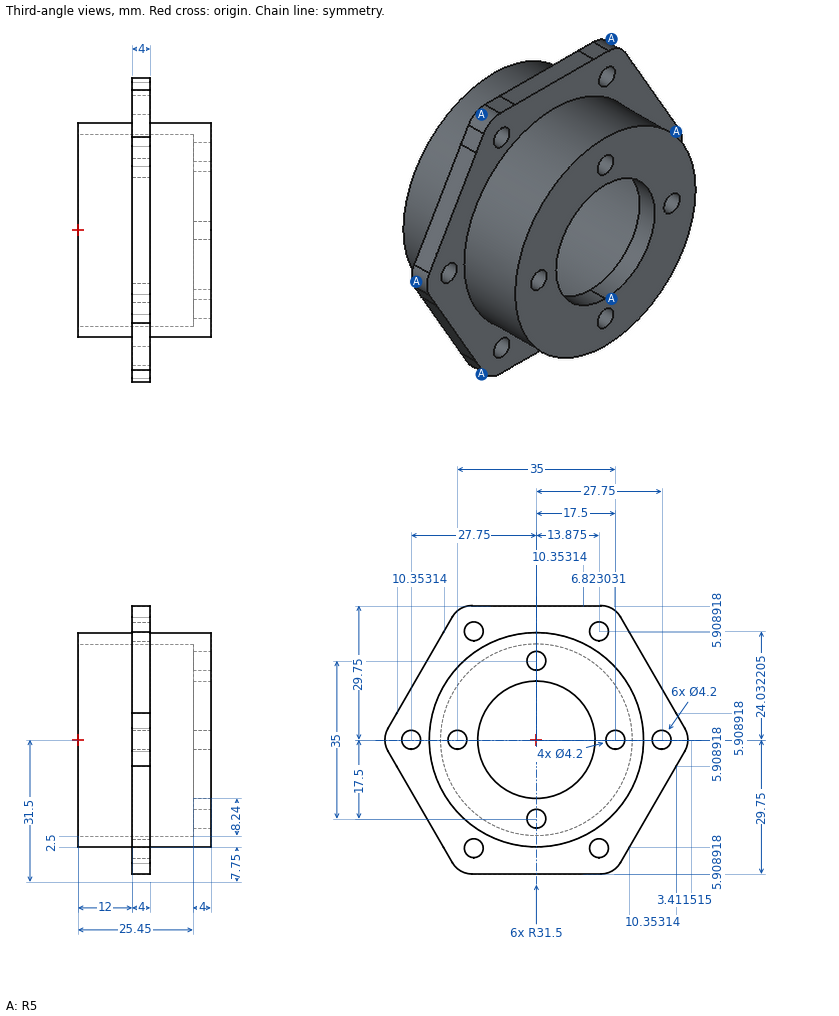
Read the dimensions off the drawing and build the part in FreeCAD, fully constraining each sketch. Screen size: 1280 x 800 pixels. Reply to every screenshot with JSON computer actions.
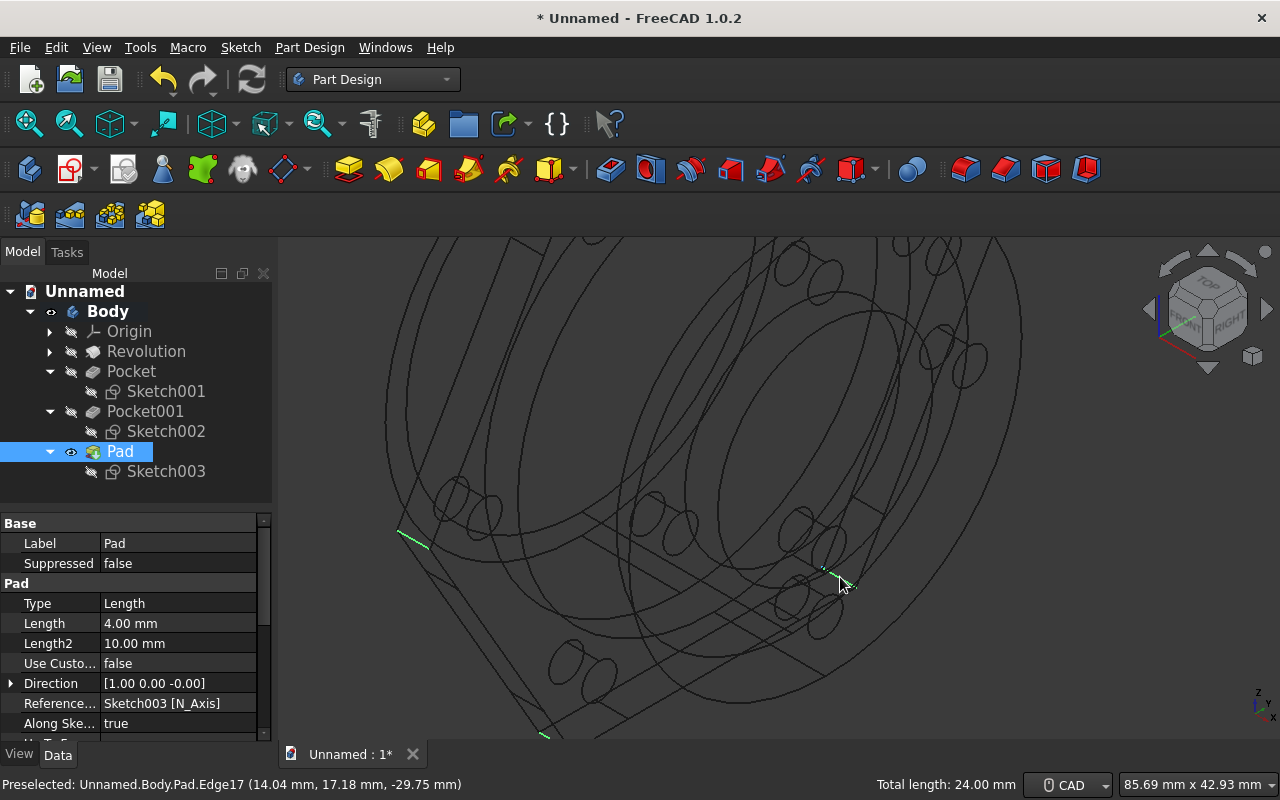
{"action": "key", "text": "v 1"}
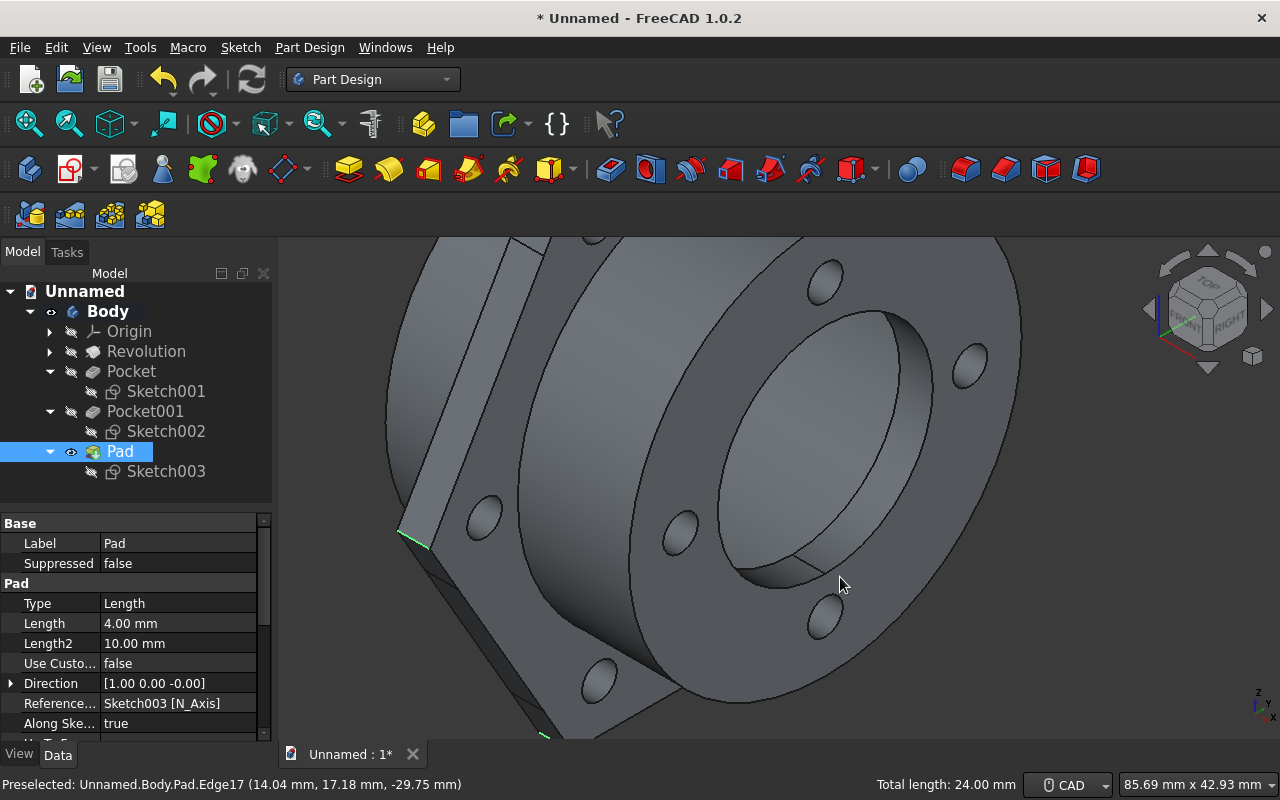
{"action": "left_click", "coordinate": [966, 170]}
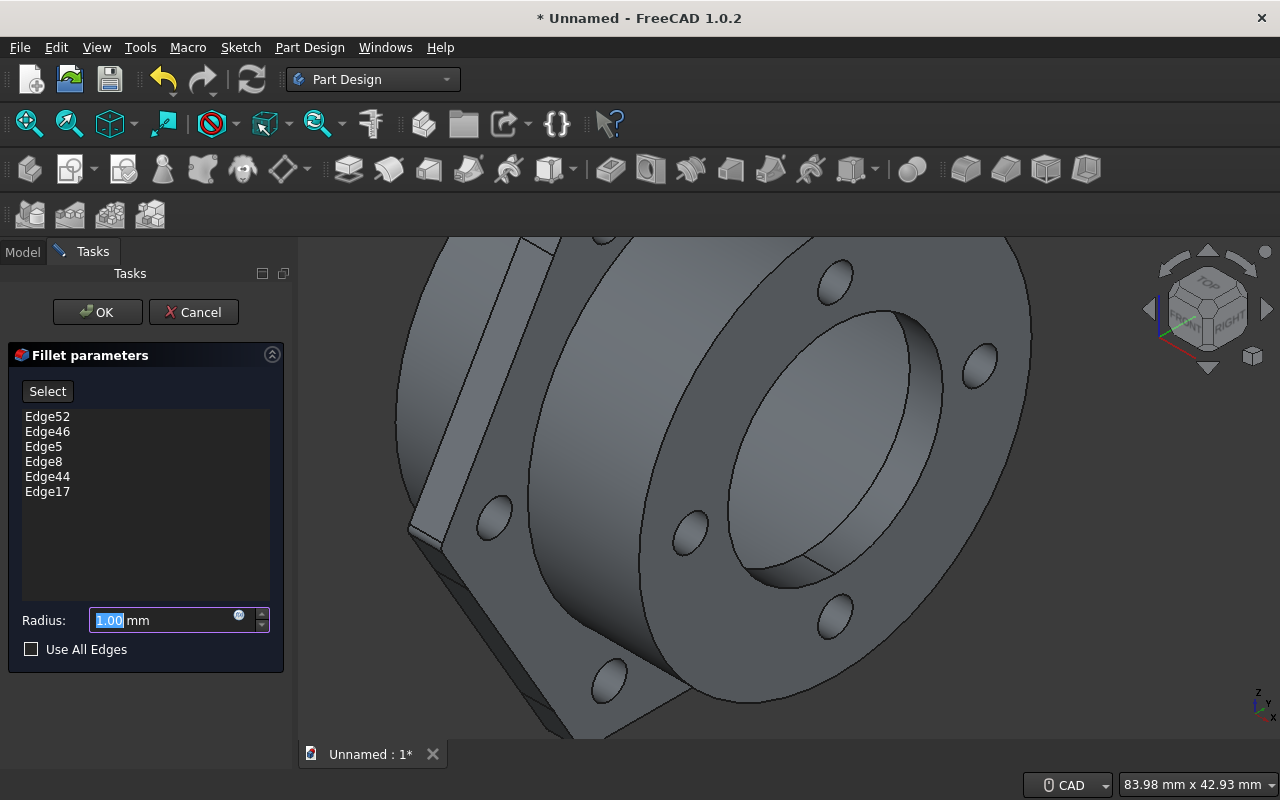
{"action": "type", "text": "5"}
{"action": "key", "text": "Tab"}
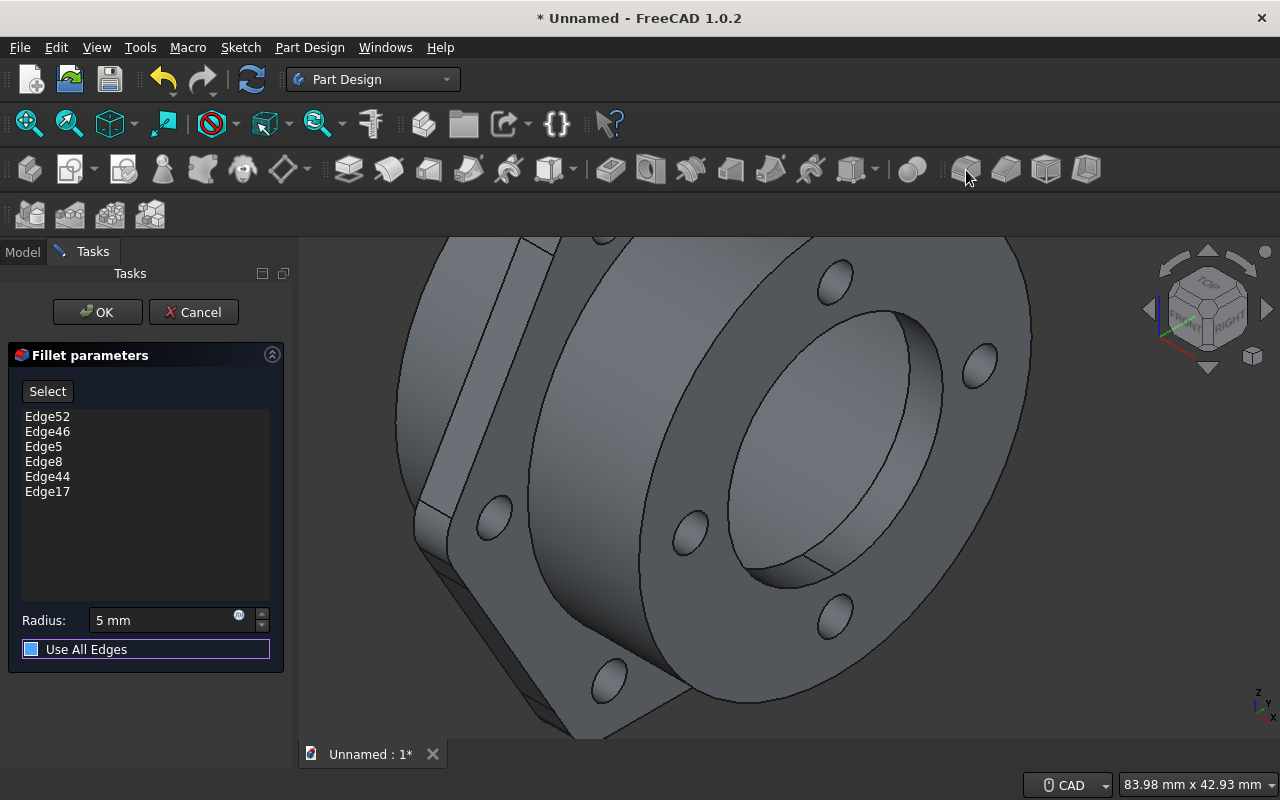
{"action": "left_click", "coordinate": [98, 312]}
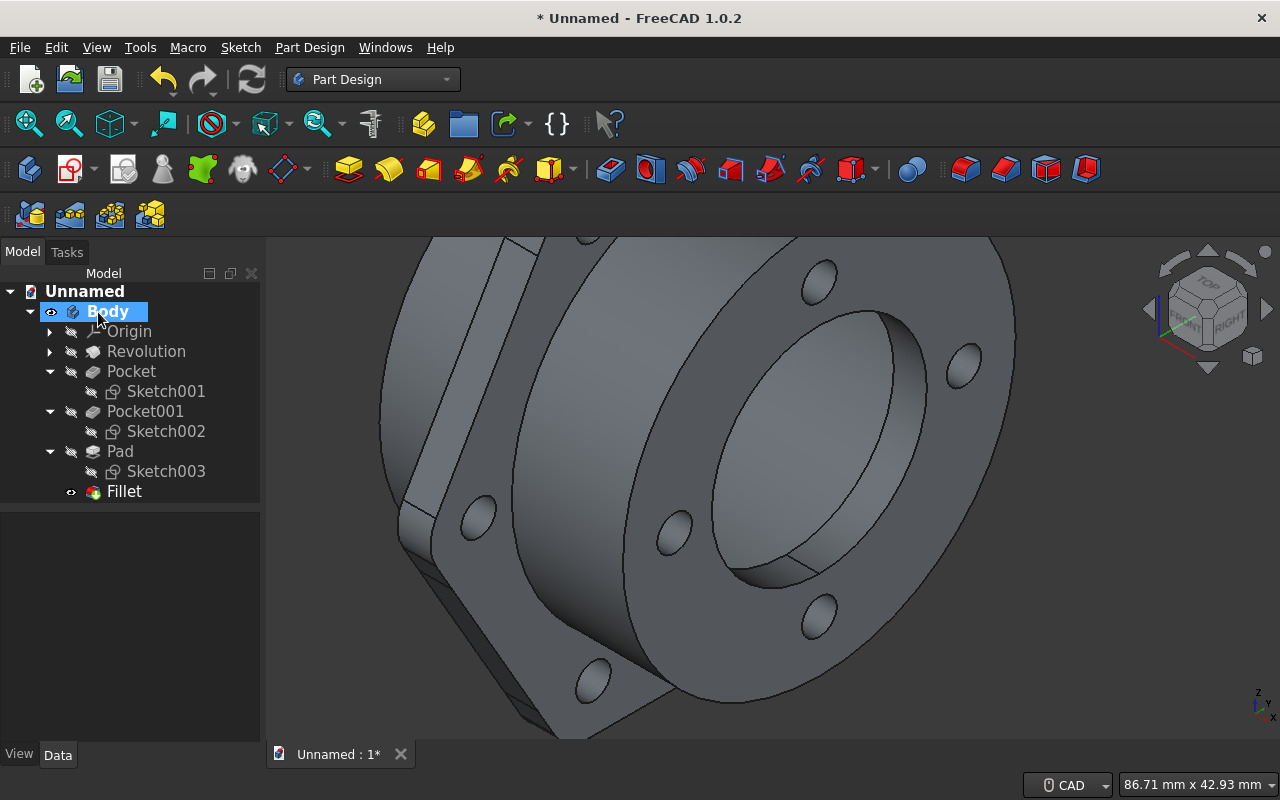
{"action": "key", "text": "v f"}